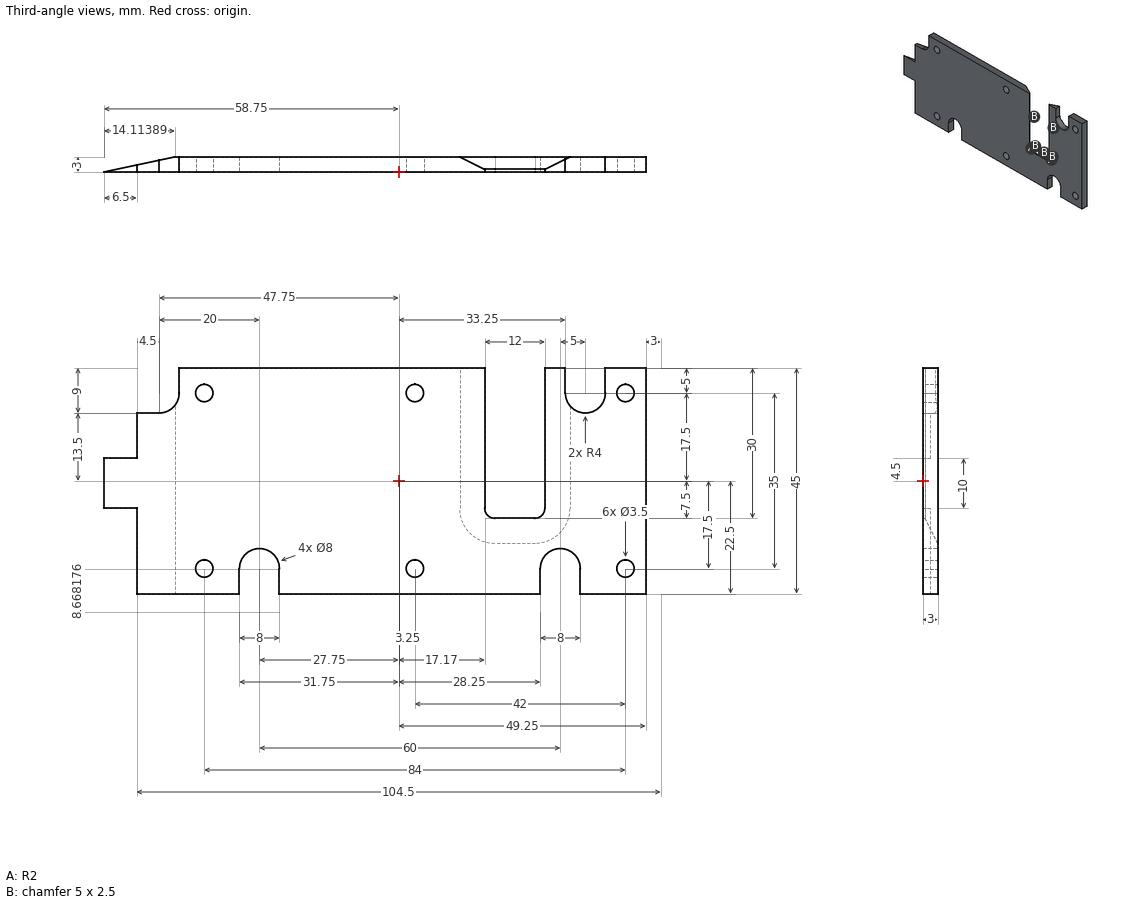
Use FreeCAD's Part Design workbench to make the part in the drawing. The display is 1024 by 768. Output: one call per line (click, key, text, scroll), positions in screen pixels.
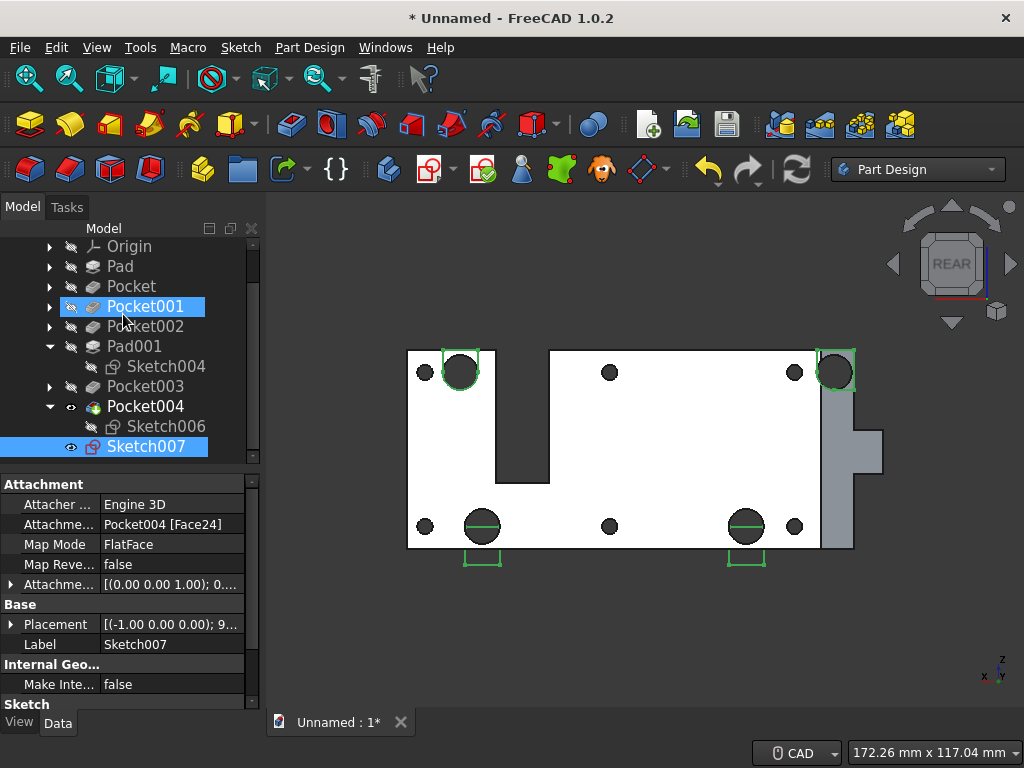
click(292, 124)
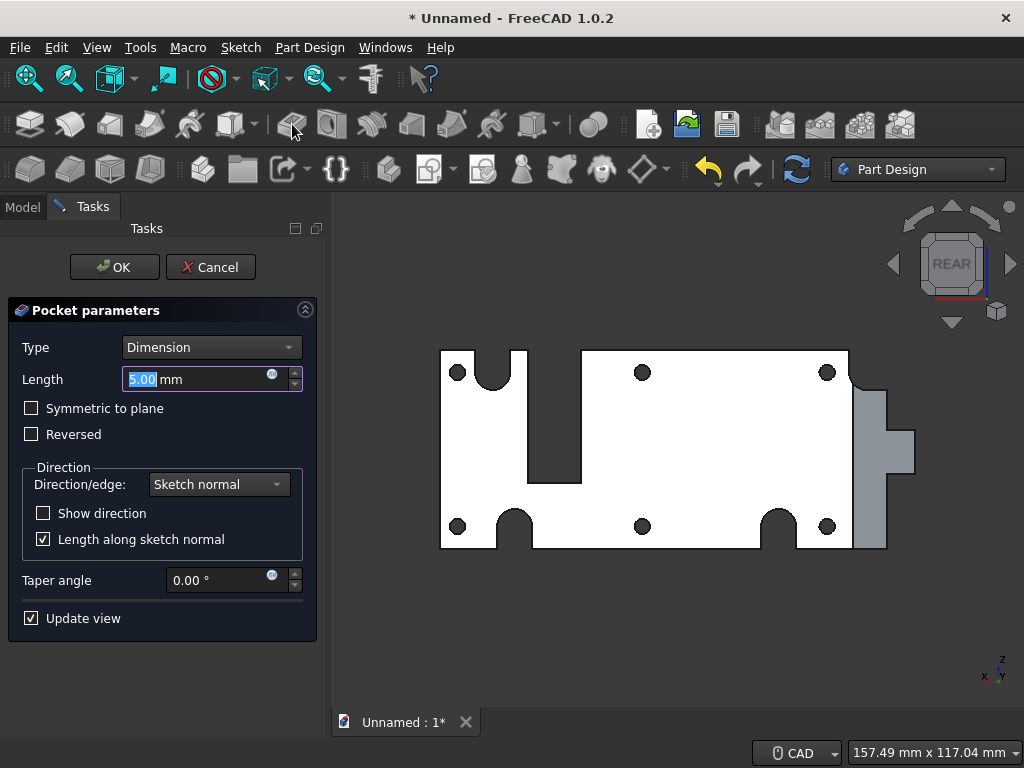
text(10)
key(Tab)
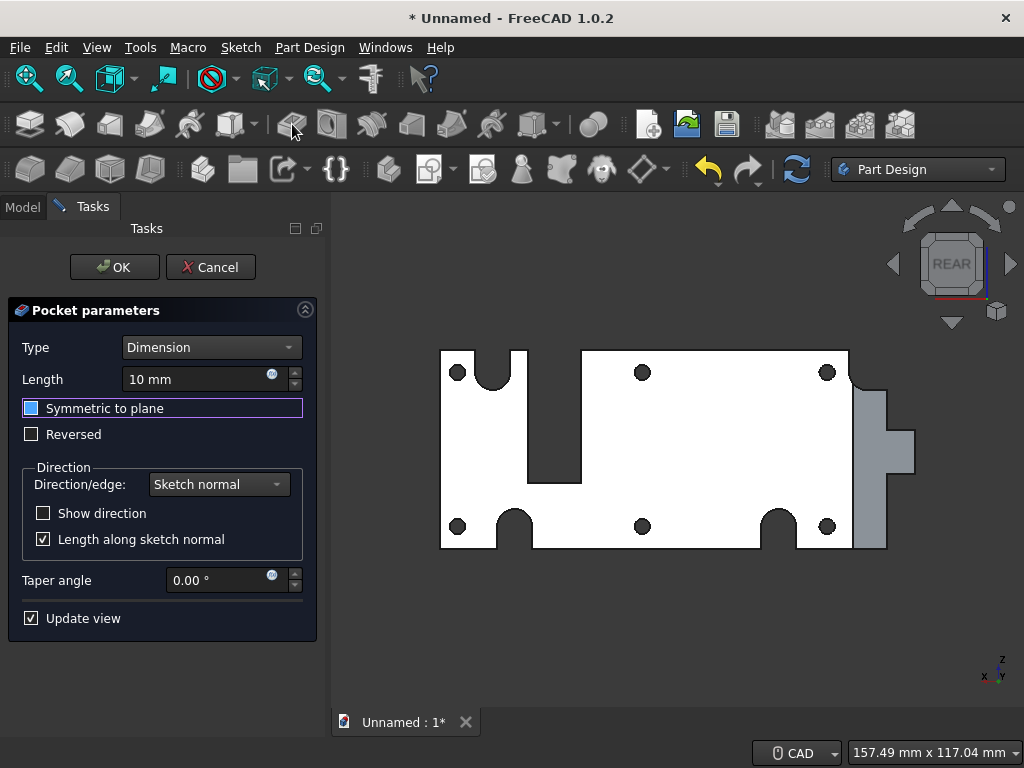
click(115, 267)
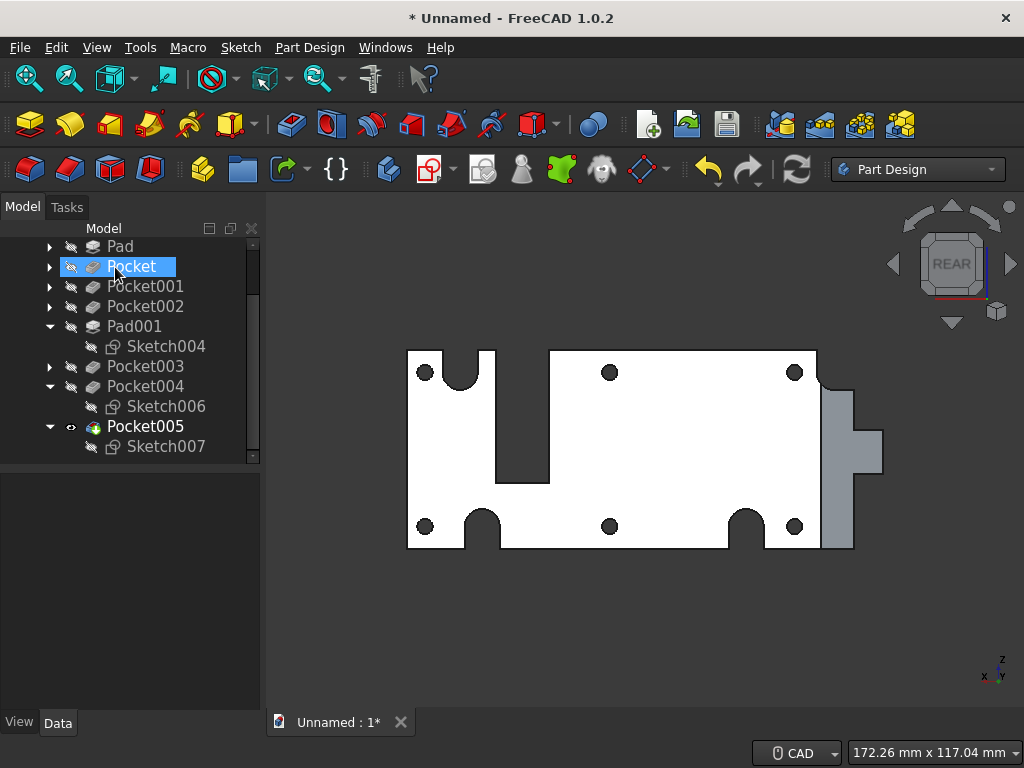
scroll(496, 482, up, 6)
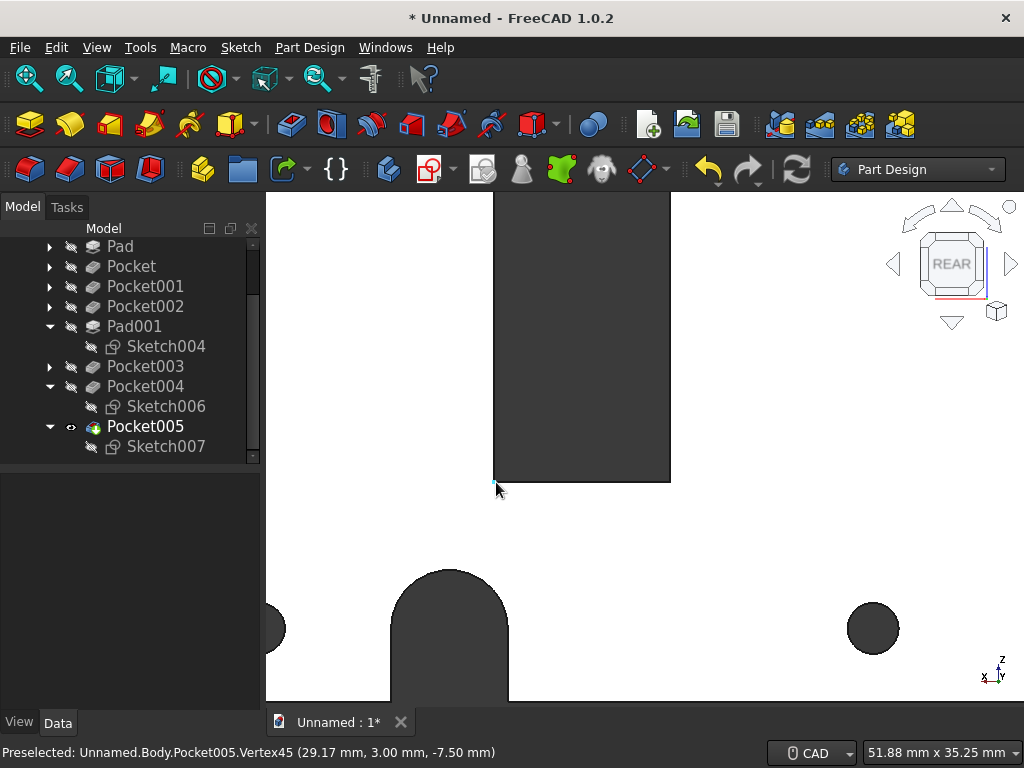
click(30, 80)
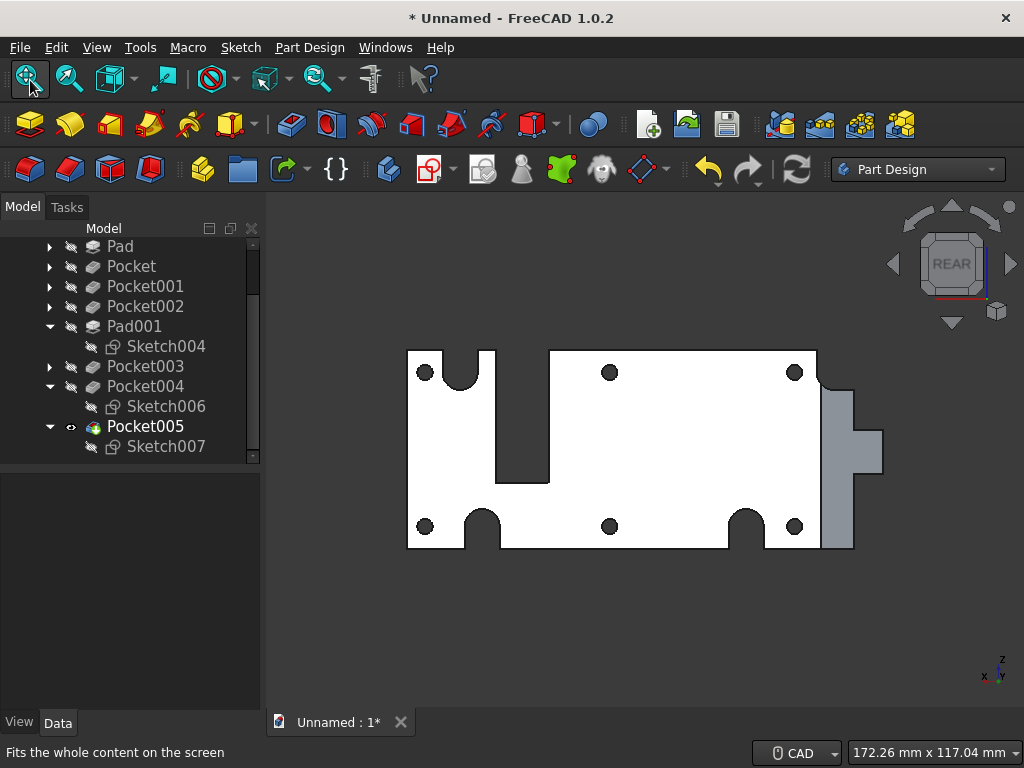
key(0)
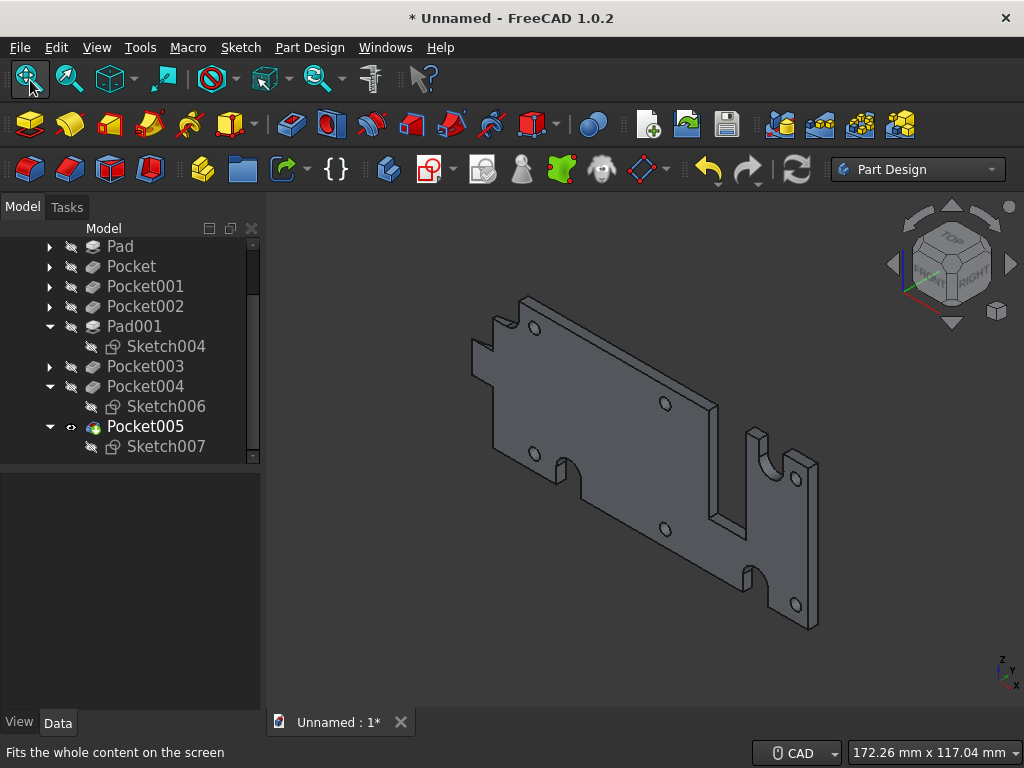
scroll(751, 536, up, 6)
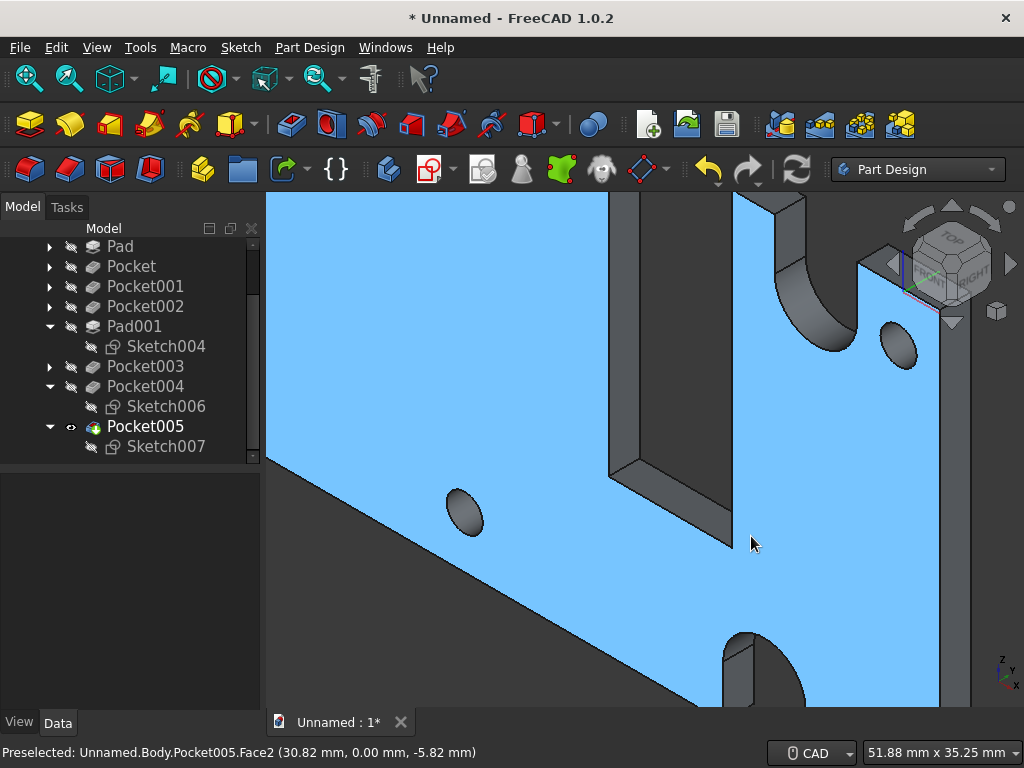
click(30, 80)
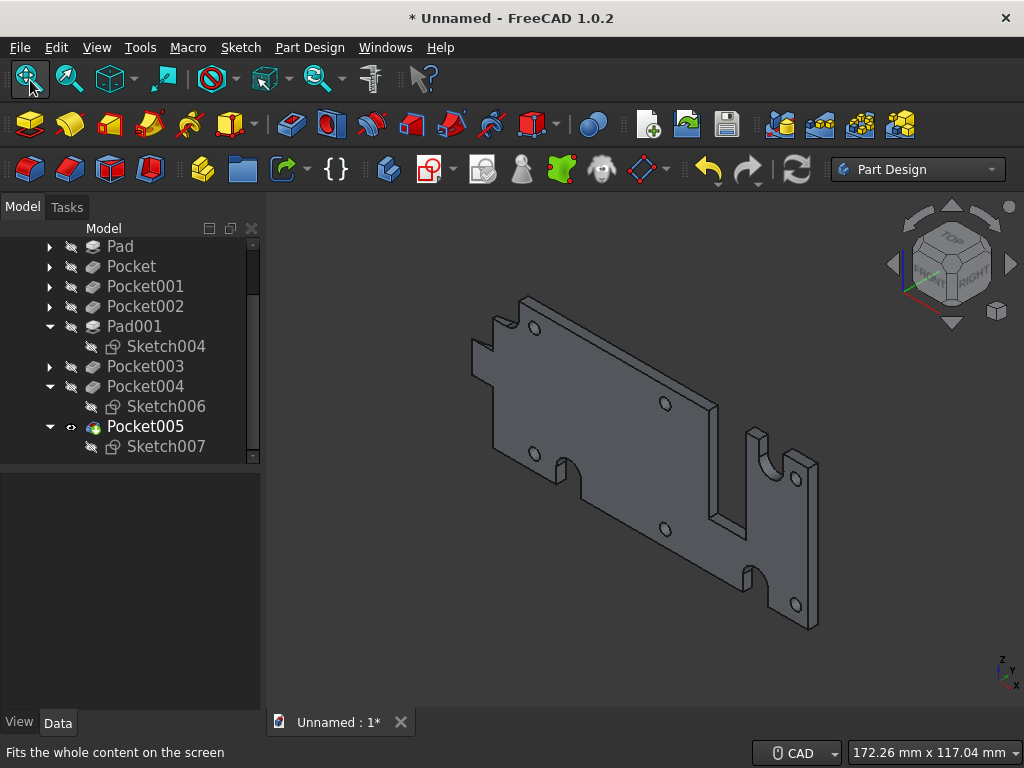
key(2)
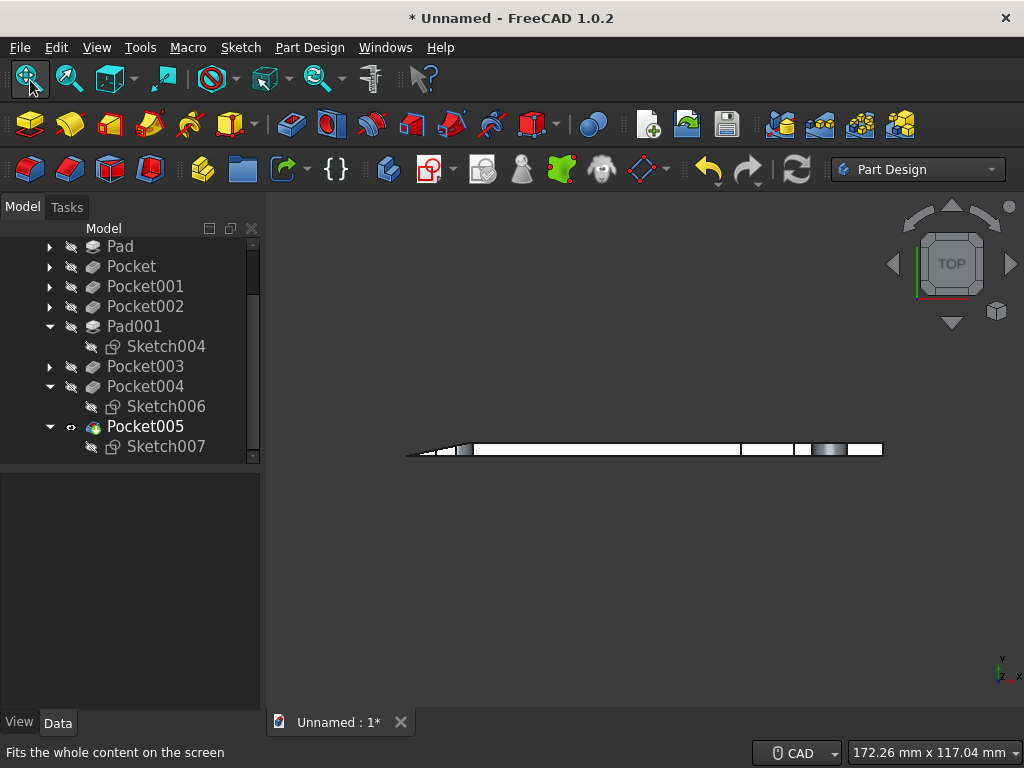
scroll(794, 448, up, 6)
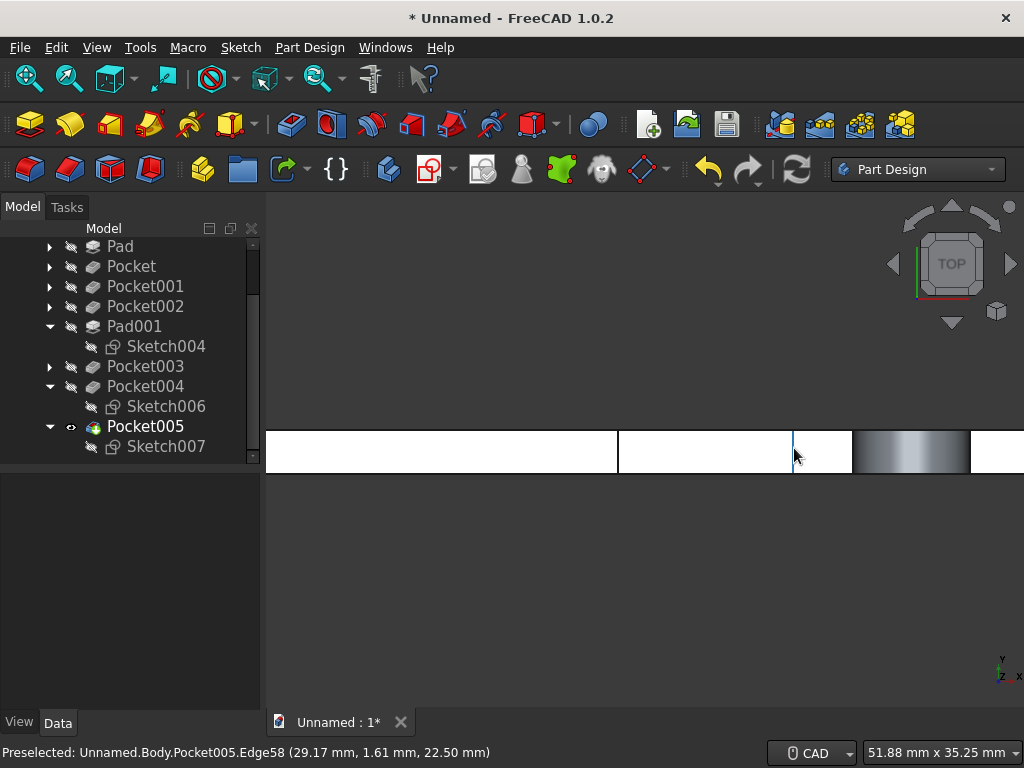
key(v)
key(f)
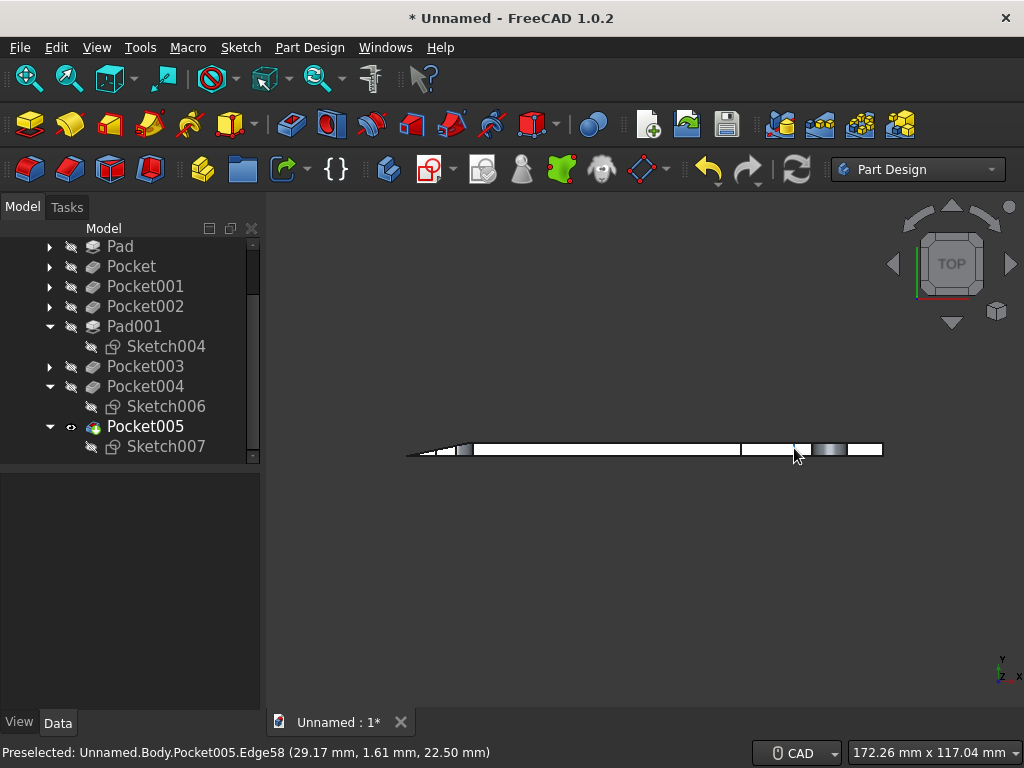
key(1)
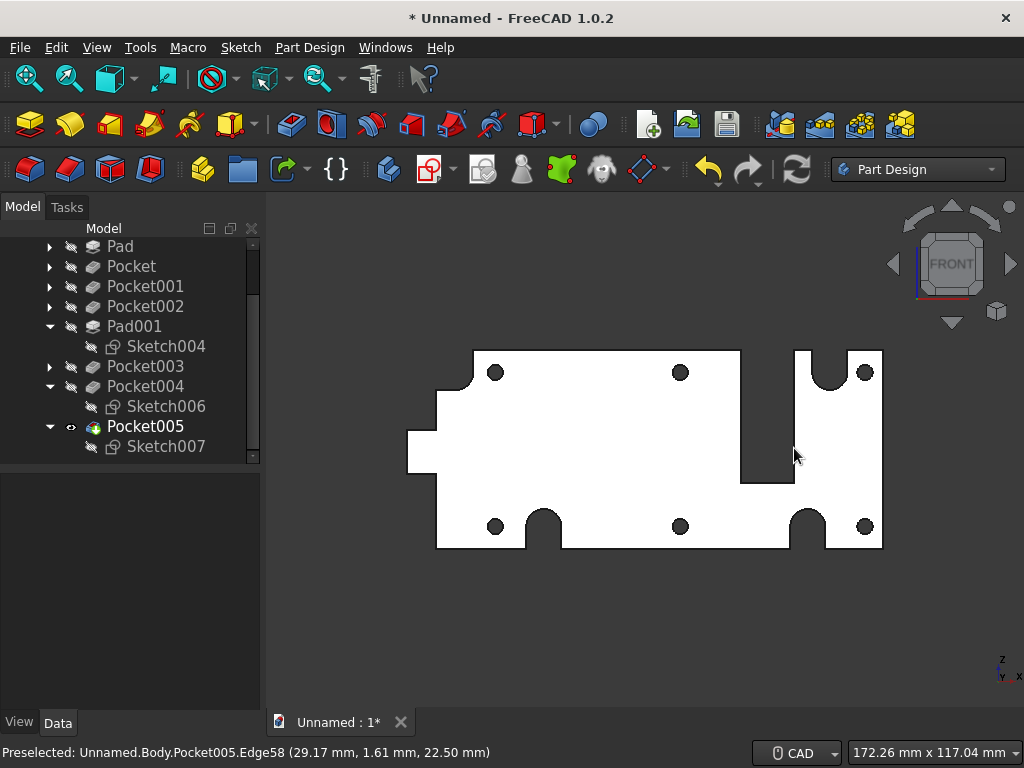
scroll(794, 482, up, 6)